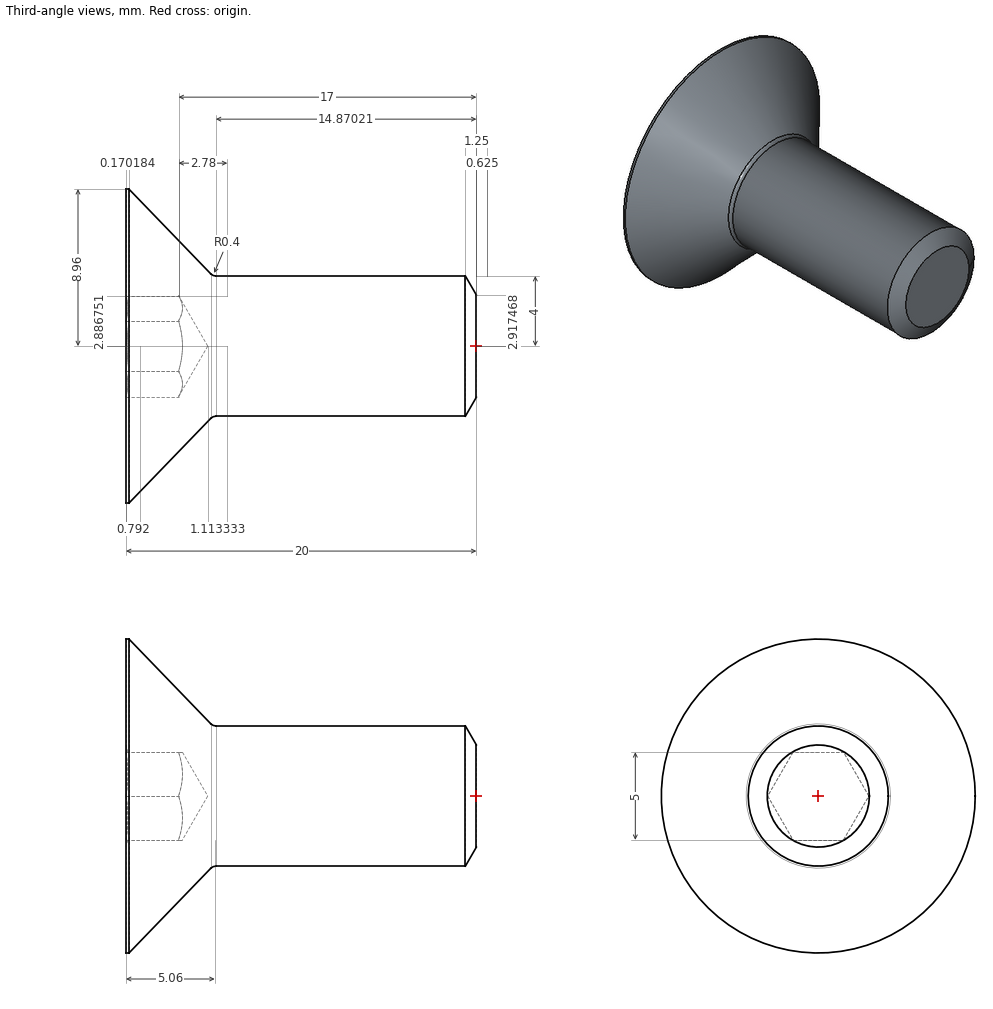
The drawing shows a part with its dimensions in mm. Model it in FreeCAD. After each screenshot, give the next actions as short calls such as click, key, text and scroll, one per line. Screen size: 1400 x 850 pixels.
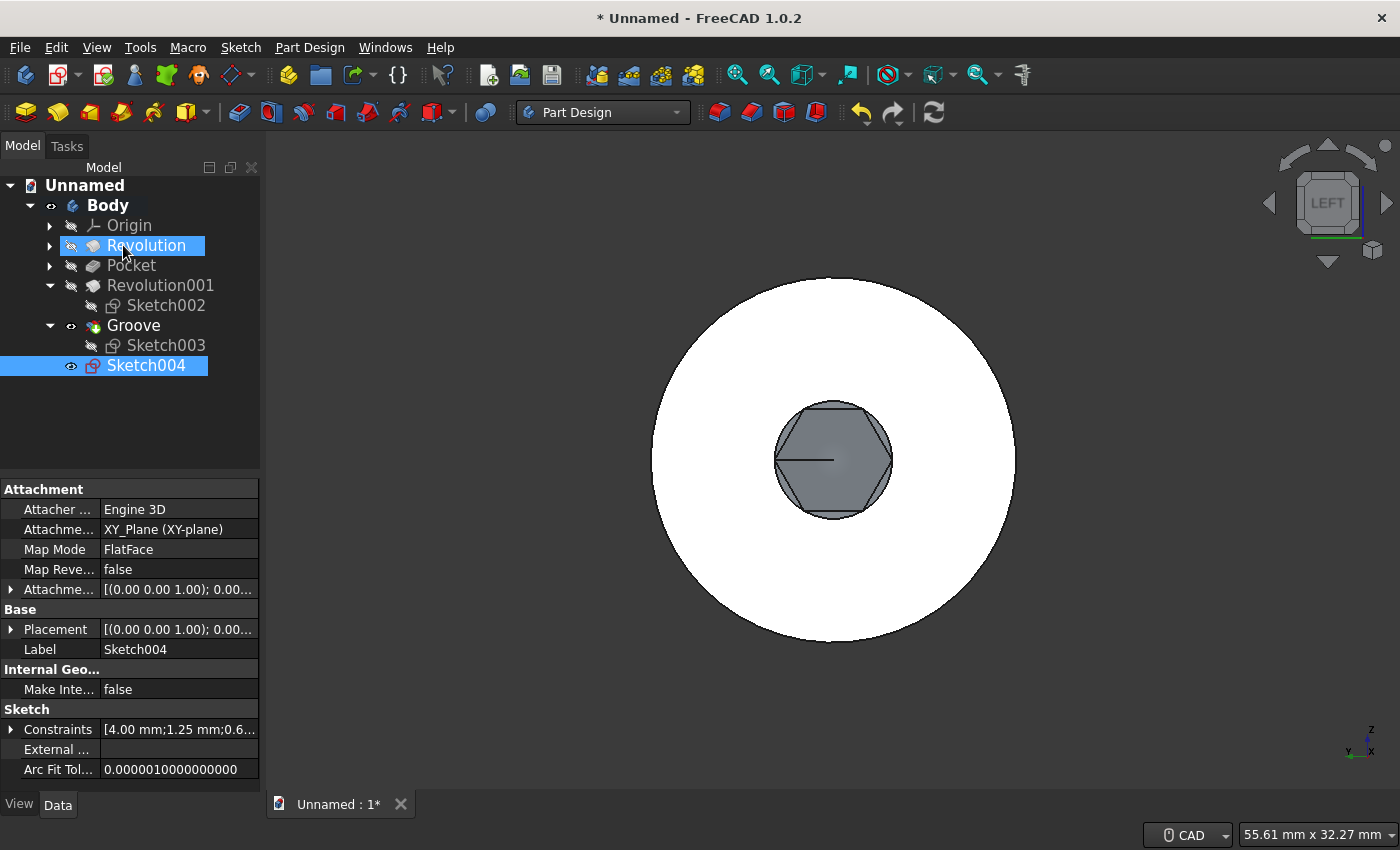
click(304, 112)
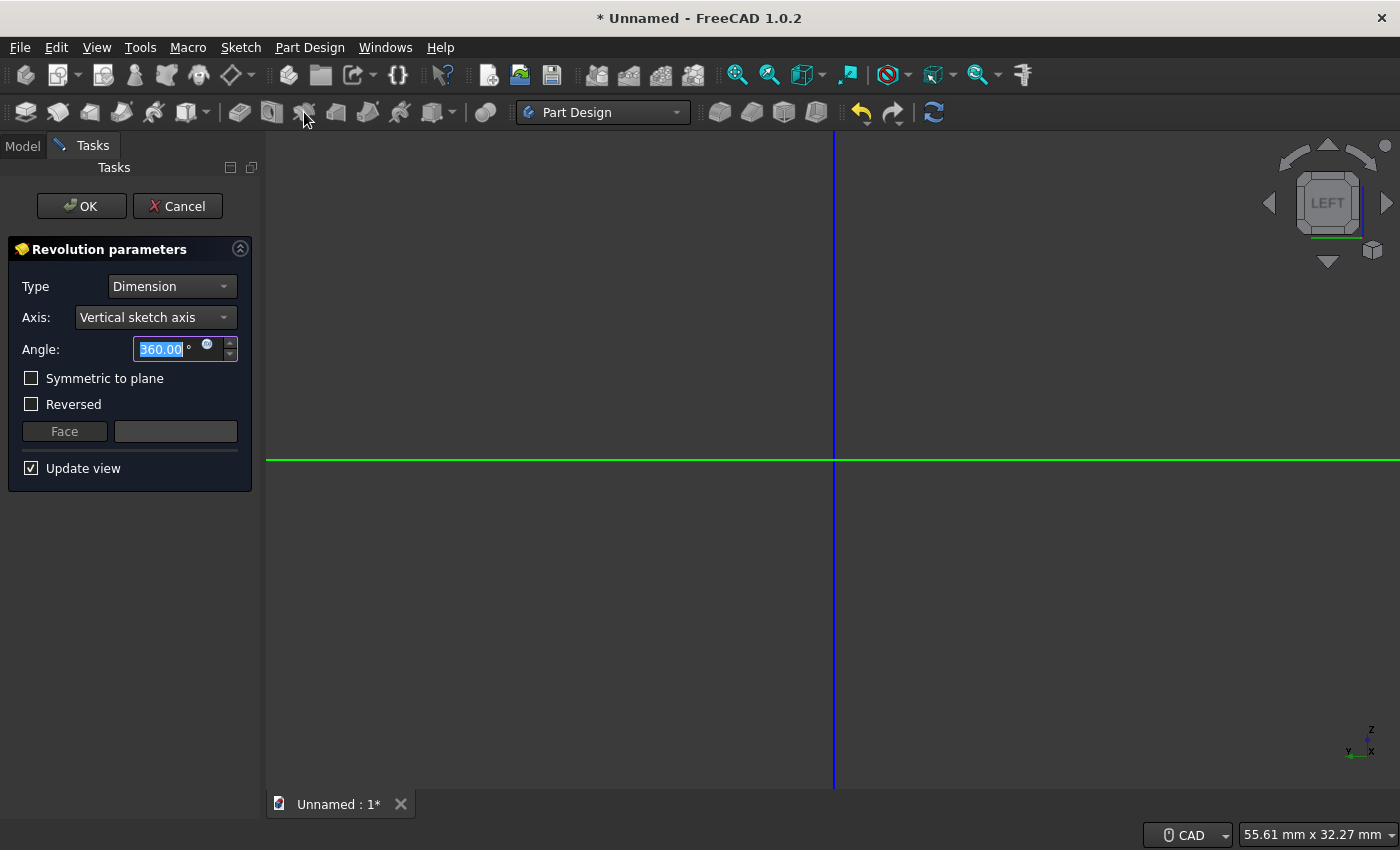
click(156, 318)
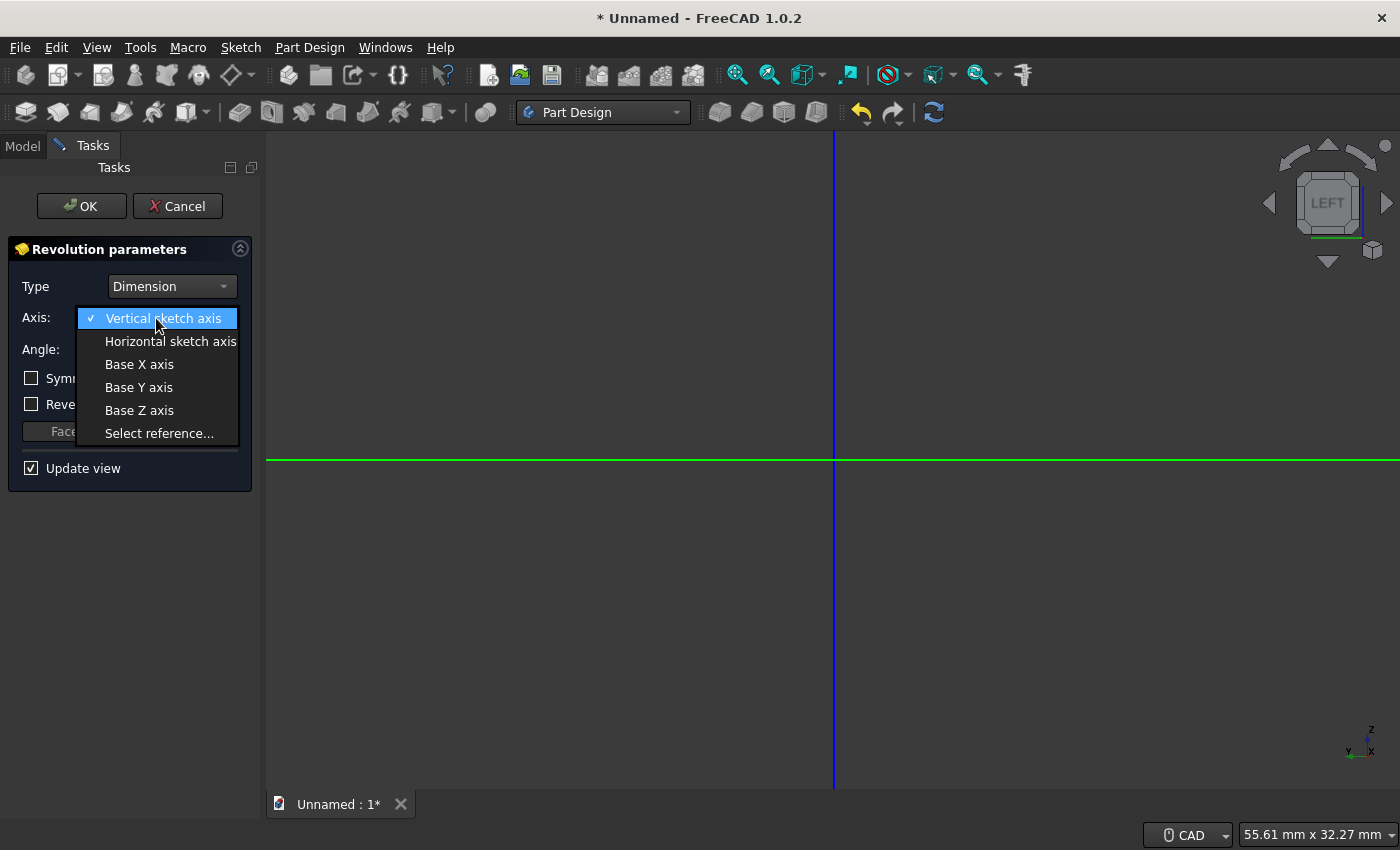
click(156, 342)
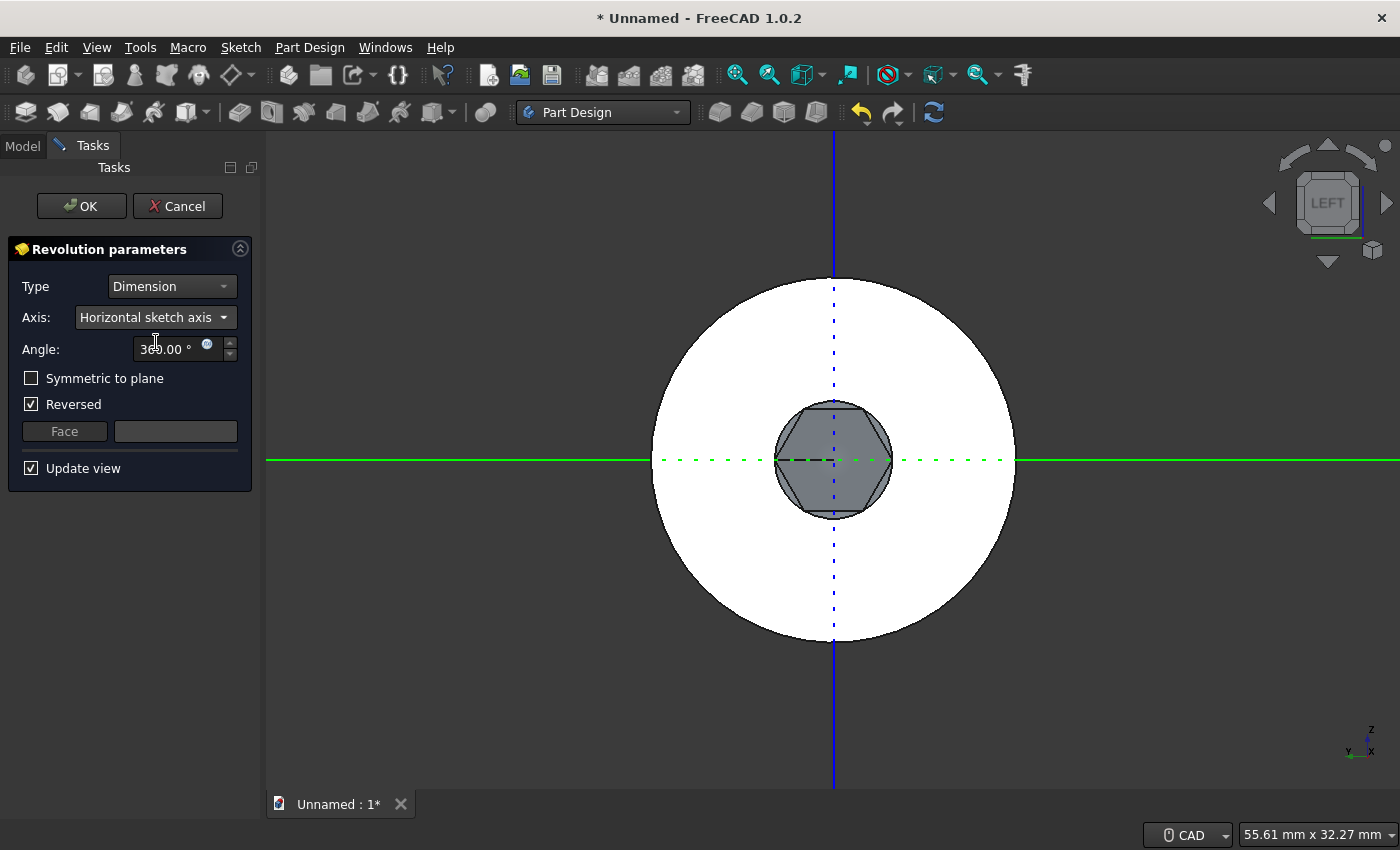
click(82, 206)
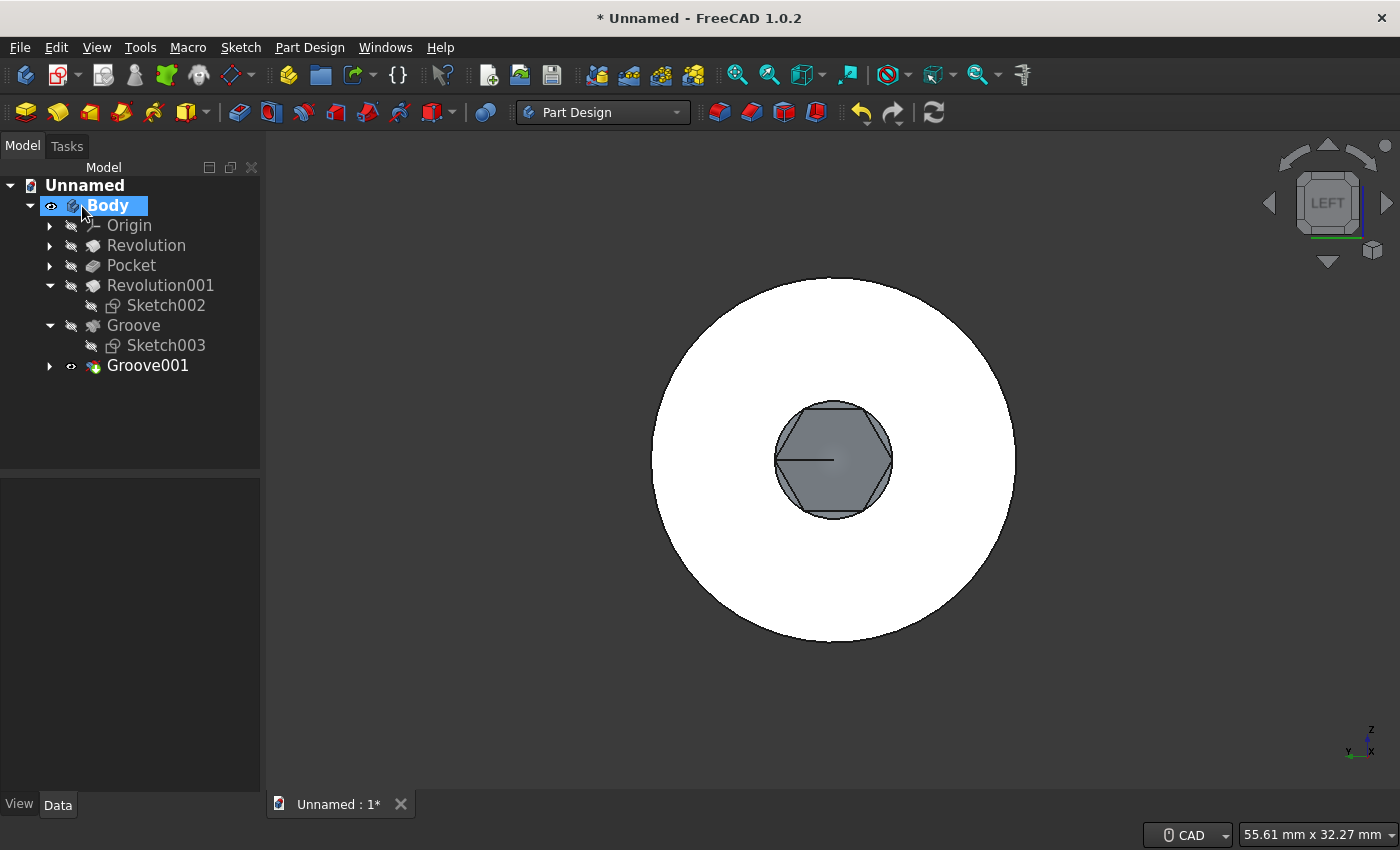
key(0)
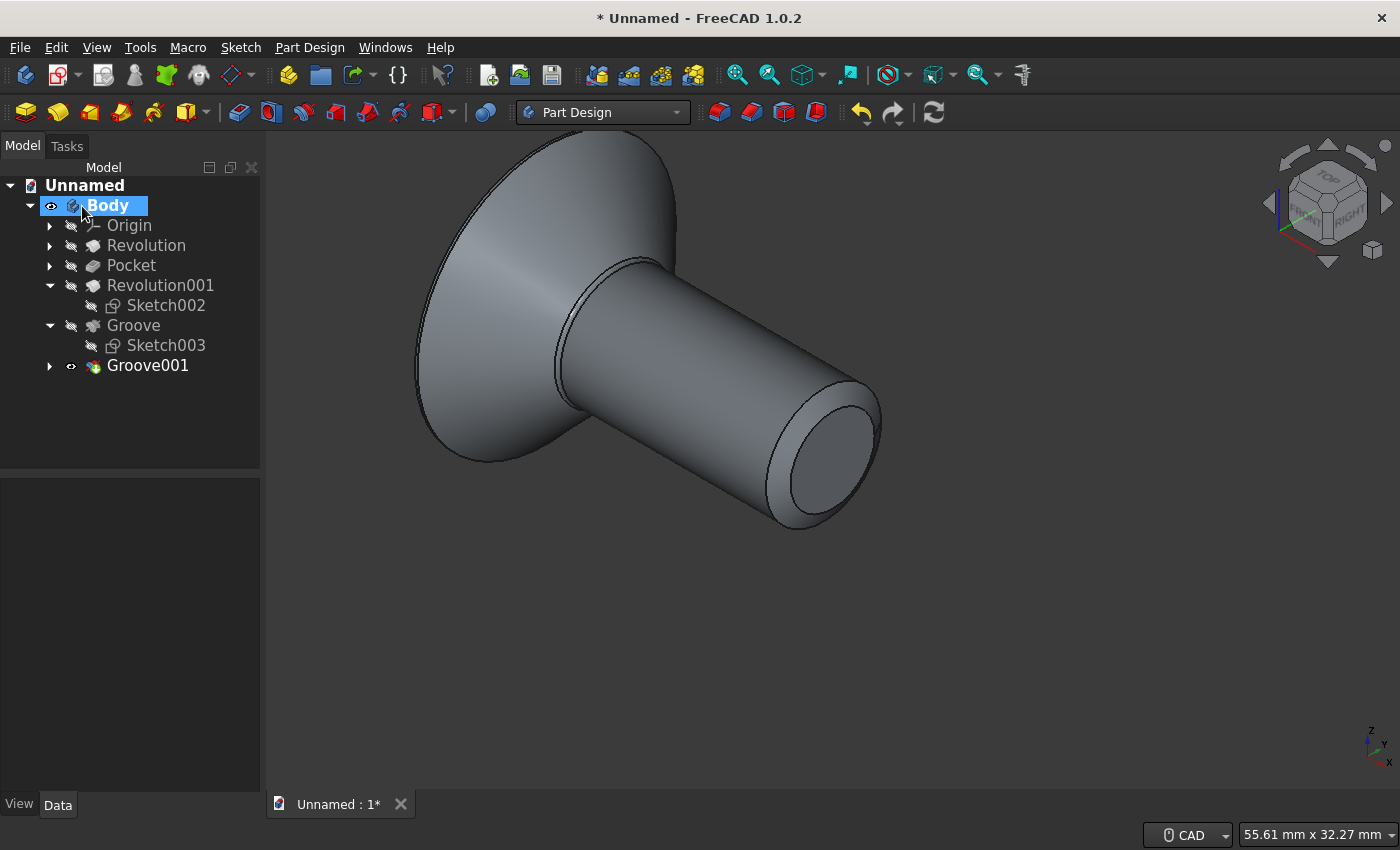
click(738, 76)